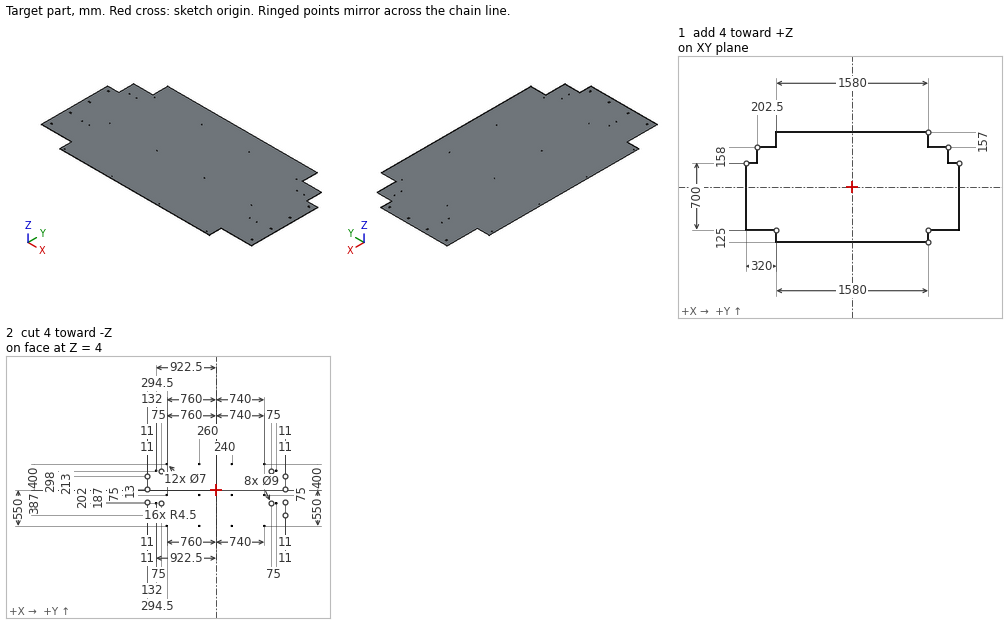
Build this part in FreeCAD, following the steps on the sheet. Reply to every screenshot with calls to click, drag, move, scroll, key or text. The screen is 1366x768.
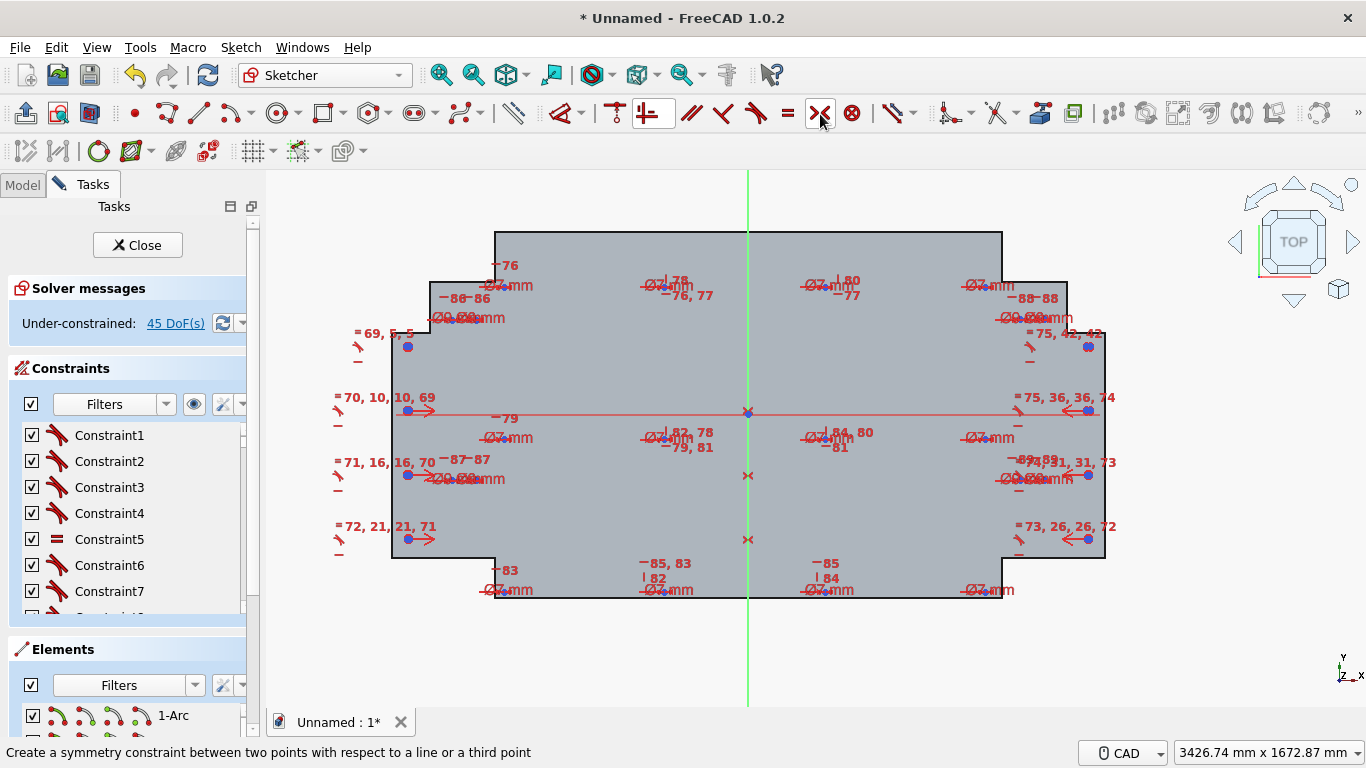
scroll(410, 347, up, 11)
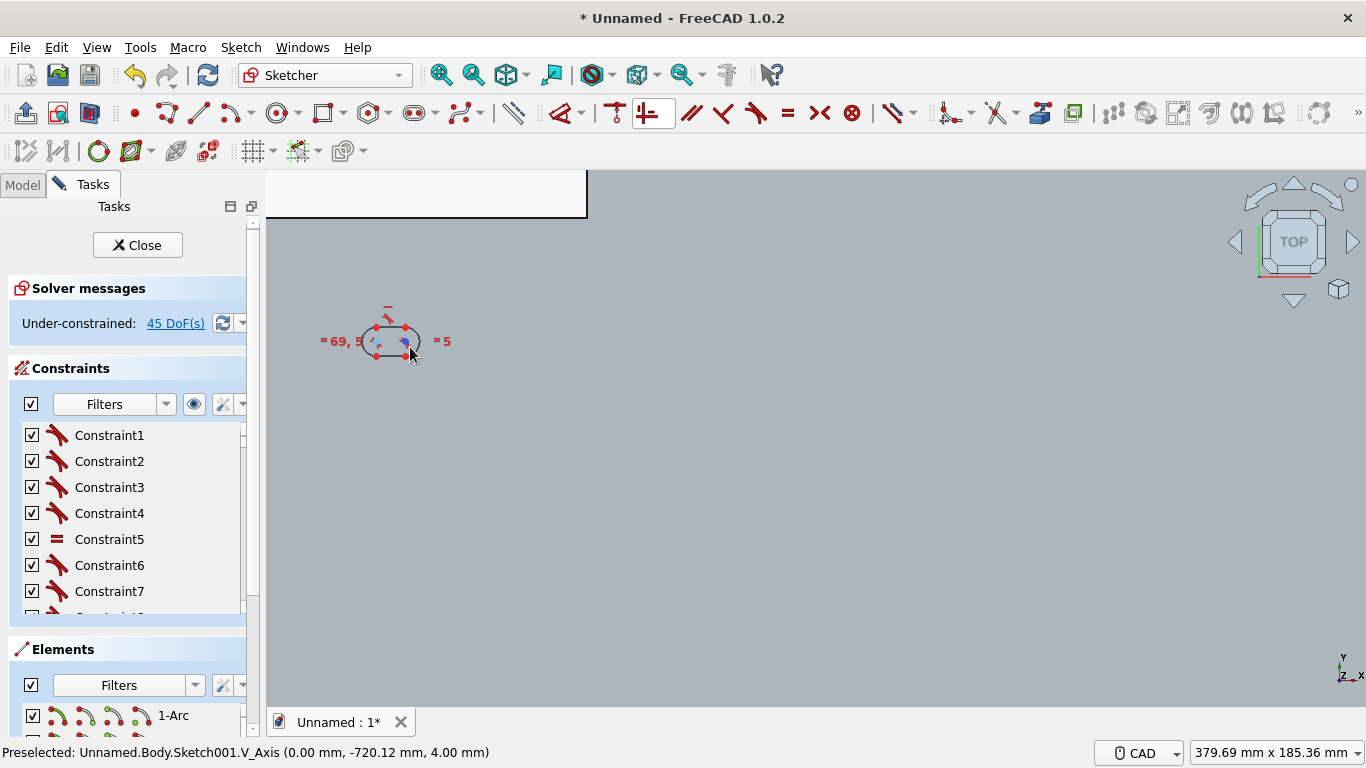
click(405, 342)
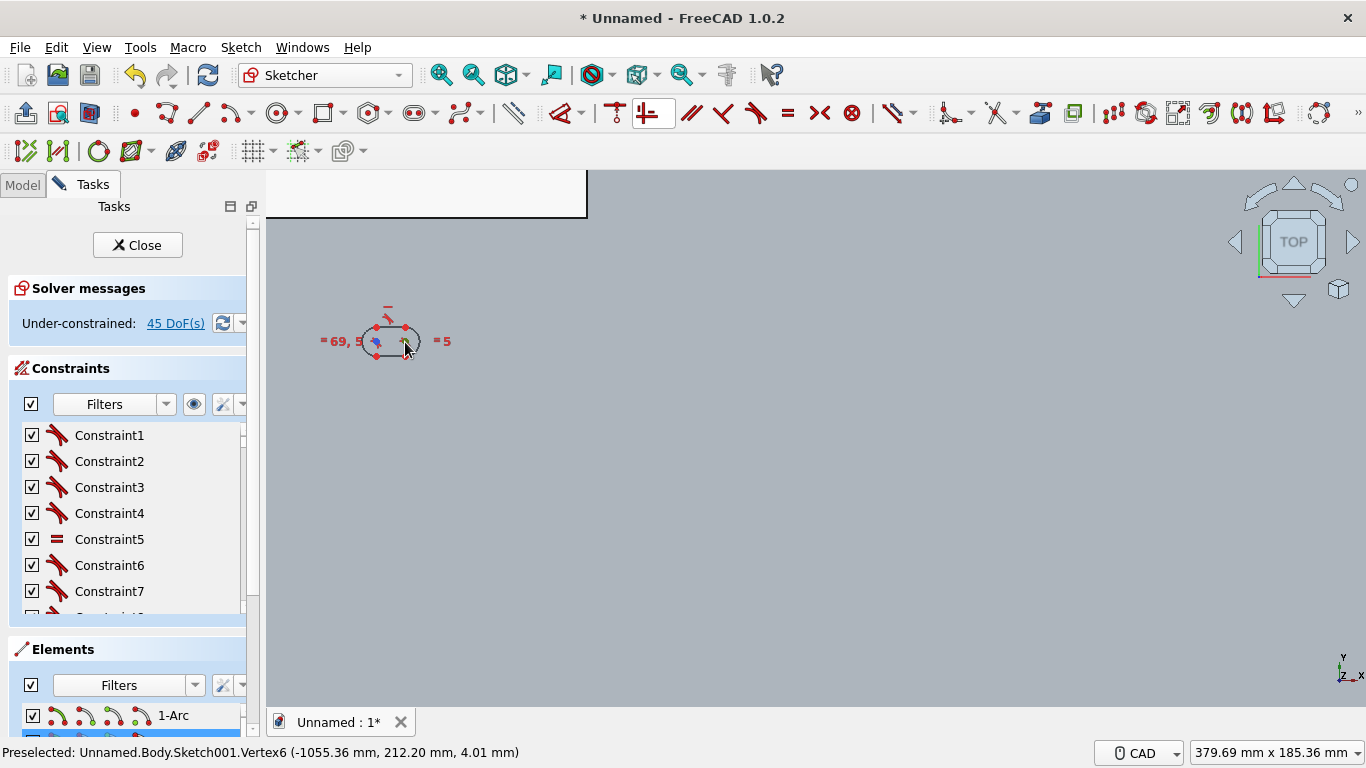
scroll(409, 347, down, 11)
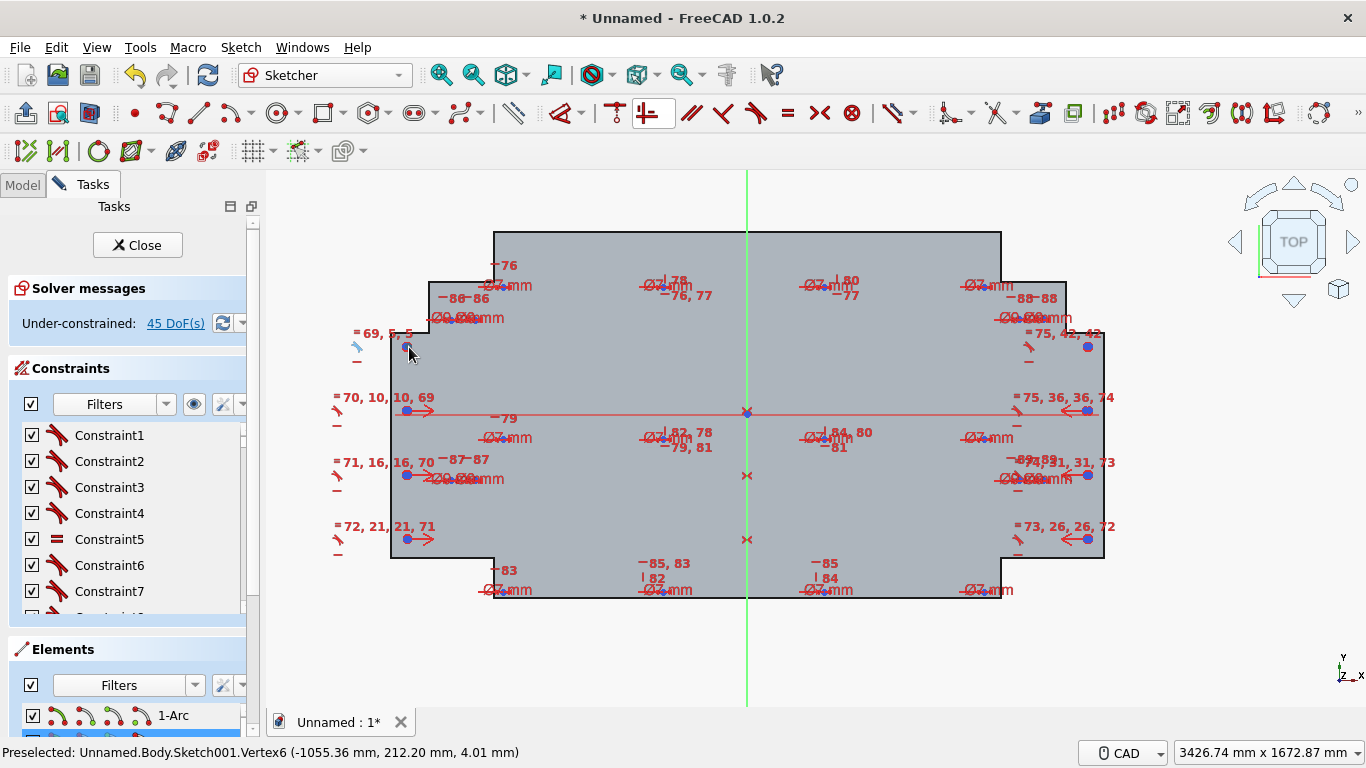
scroll(1086, 347, up, 11)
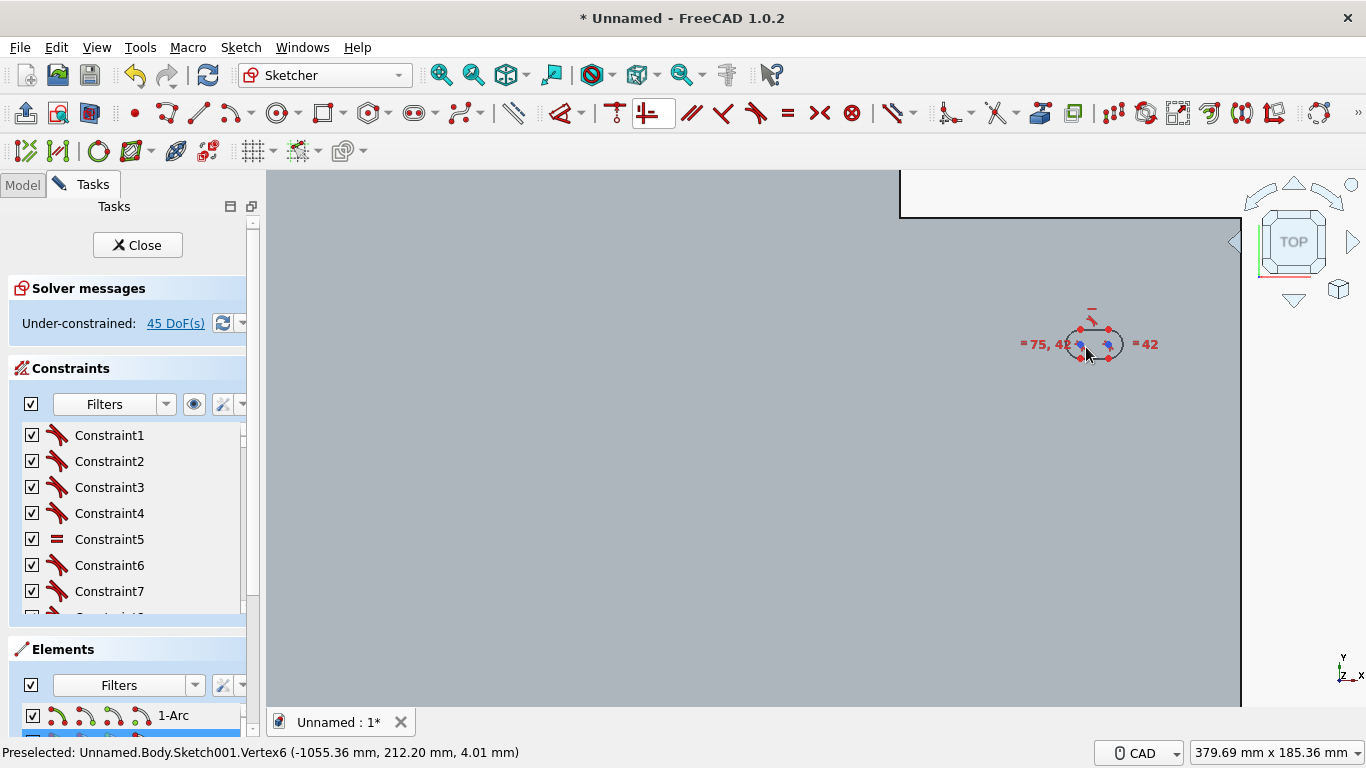
click(1081, 344)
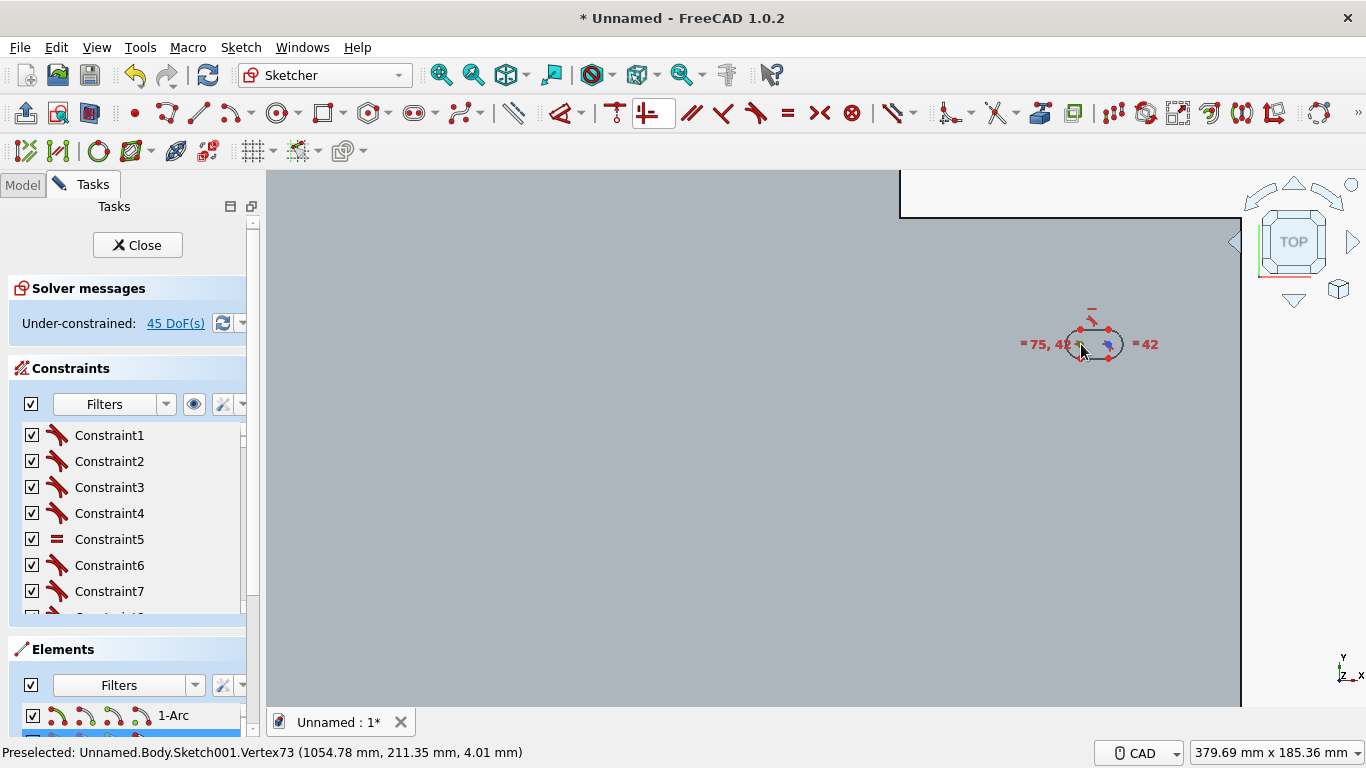
scroll(1087, 347, down, 11)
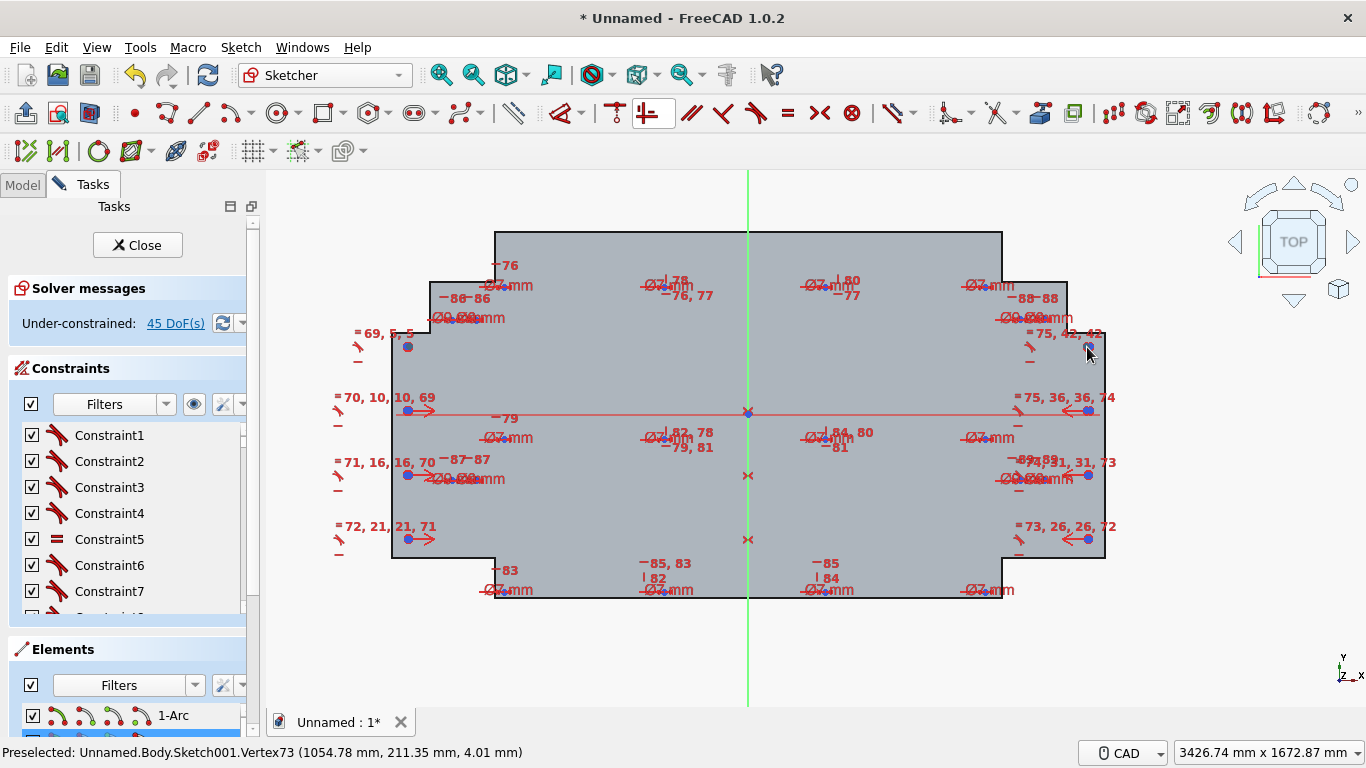
click(748, 645)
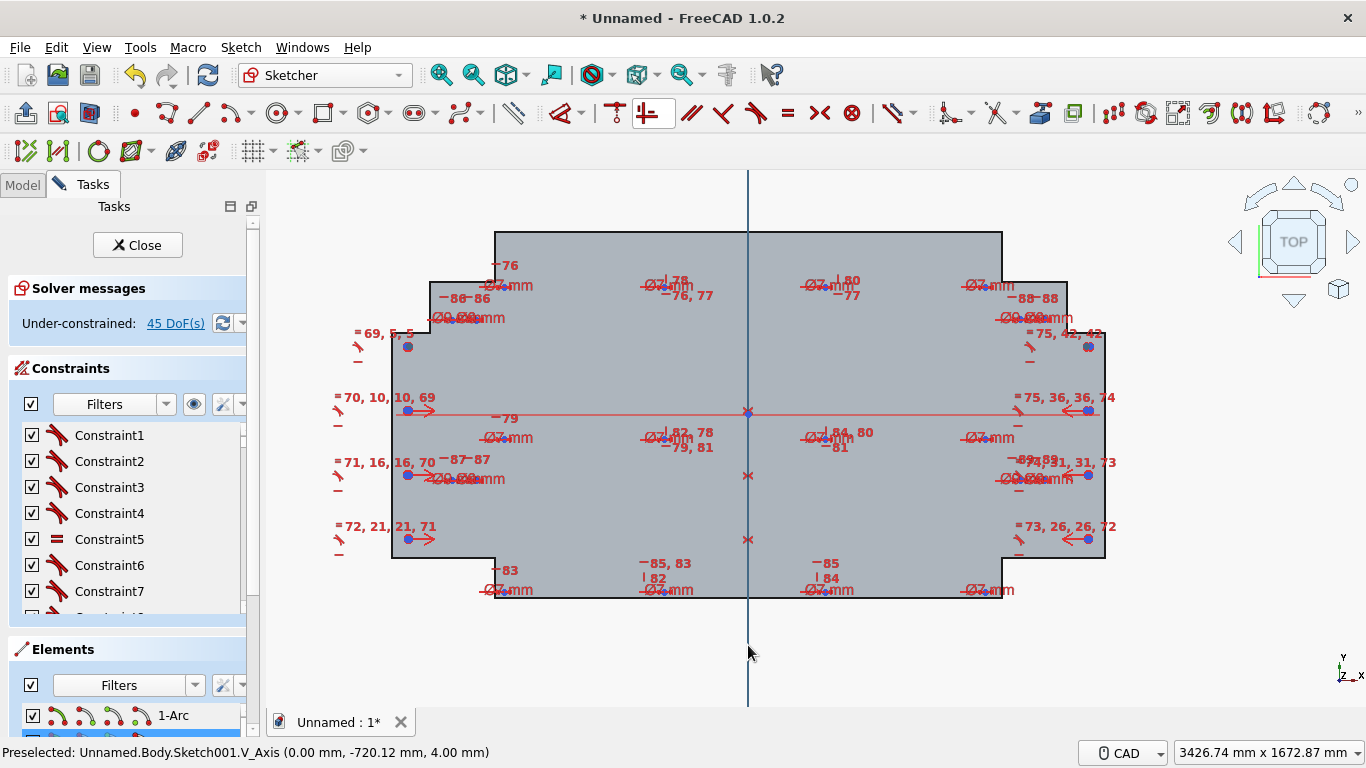
click(820, 114)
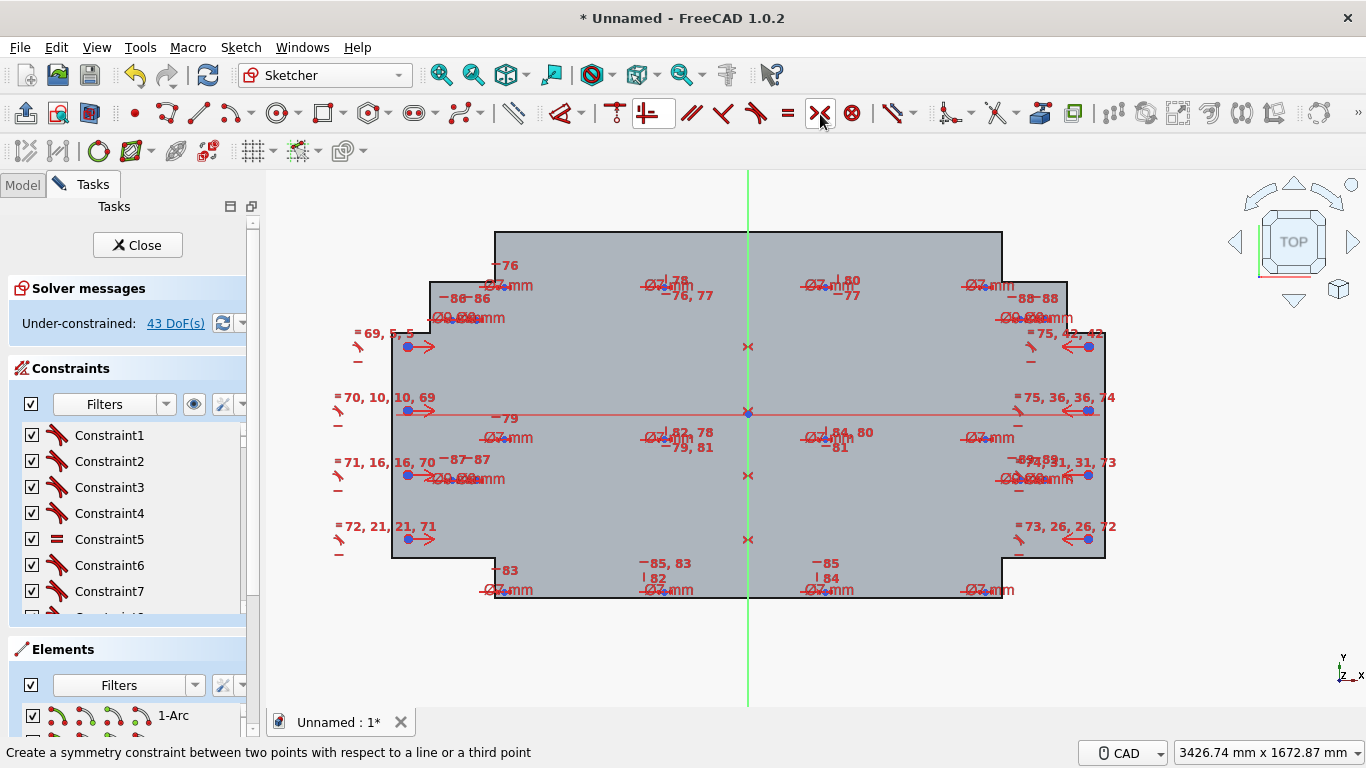
click(476, 320)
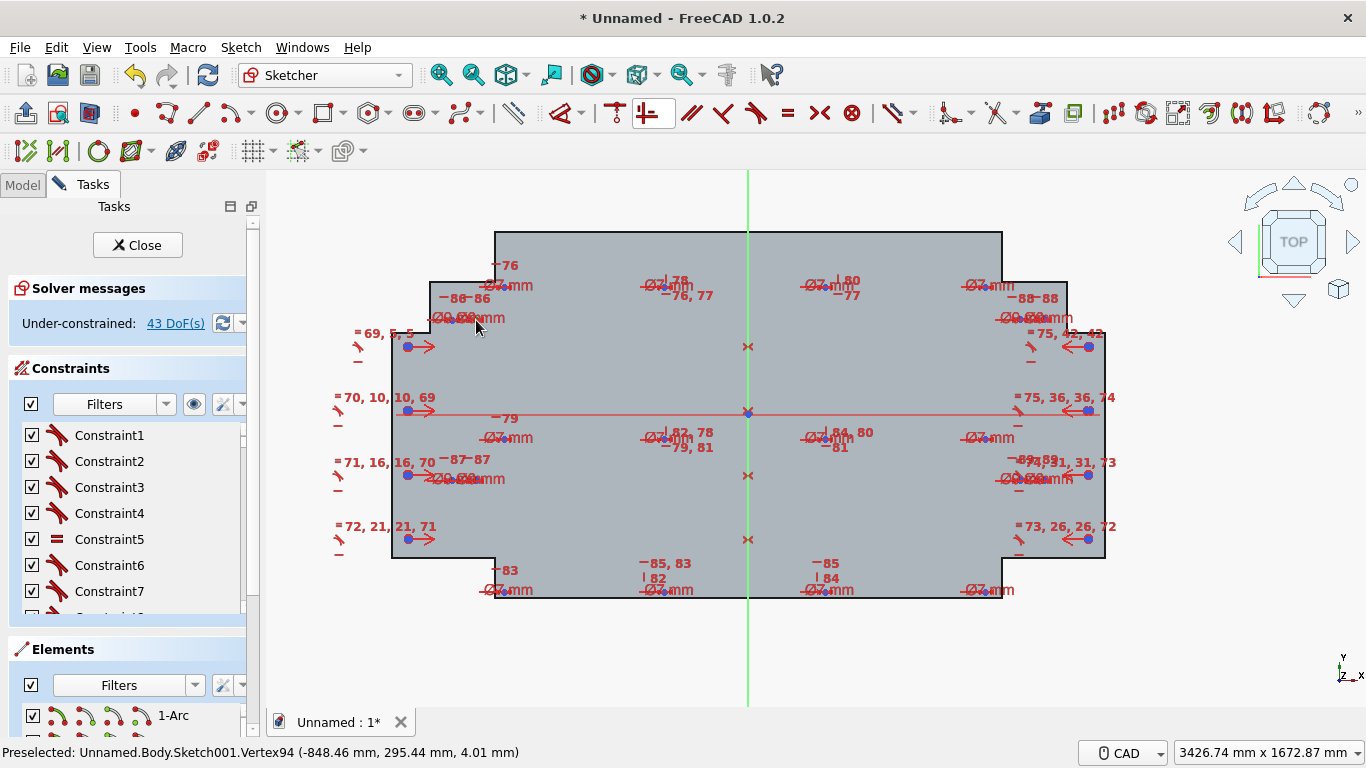
click(1020, 320)